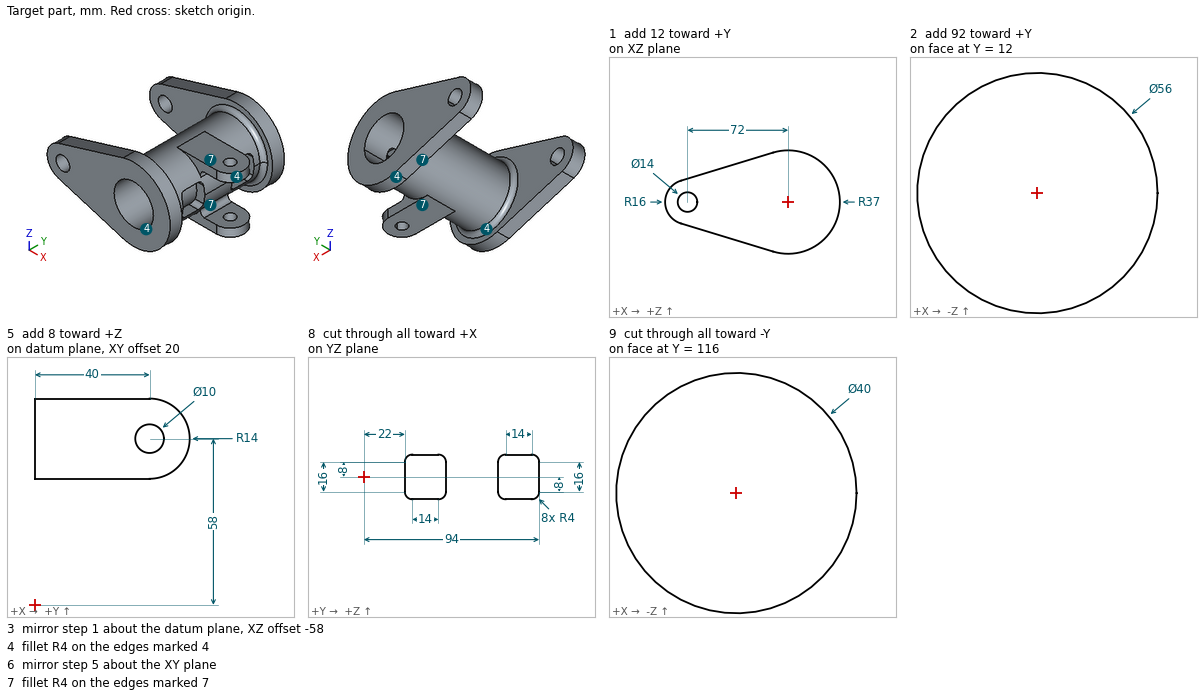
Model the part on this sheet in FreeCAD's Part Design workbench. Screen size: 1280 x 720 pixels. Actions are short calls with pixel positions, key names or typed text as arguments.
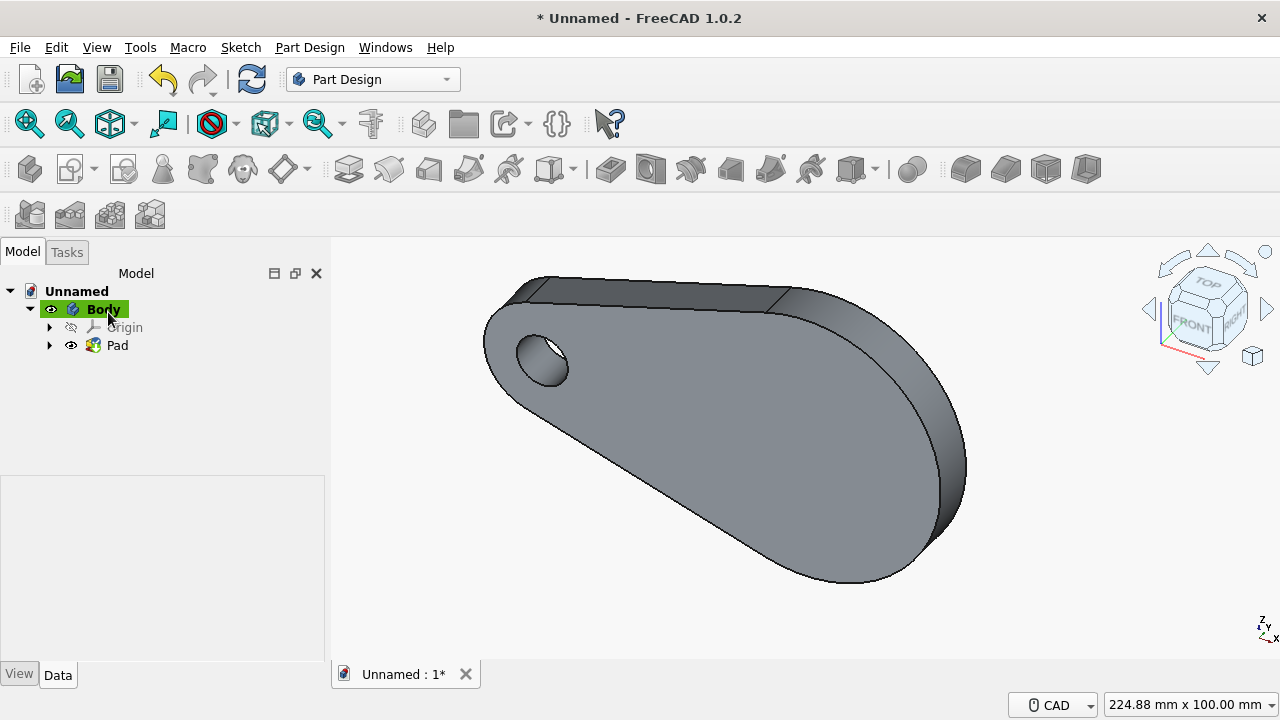
click(30, 124)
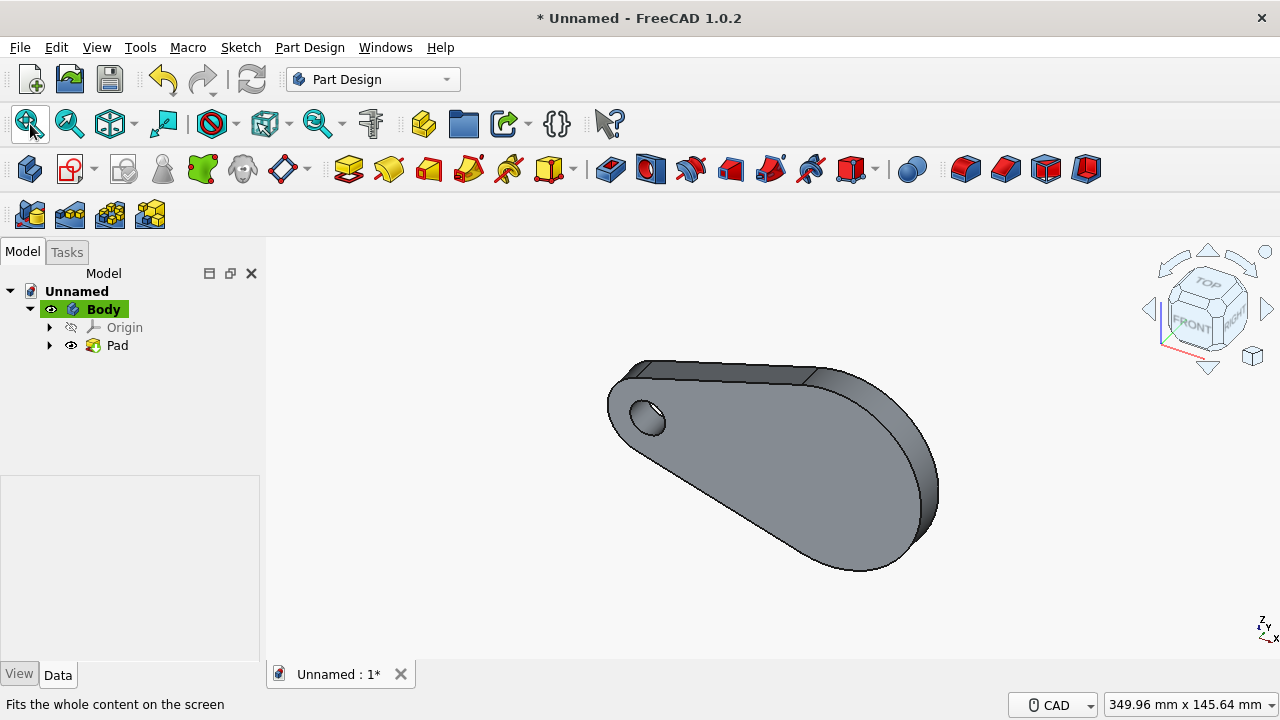
key(4)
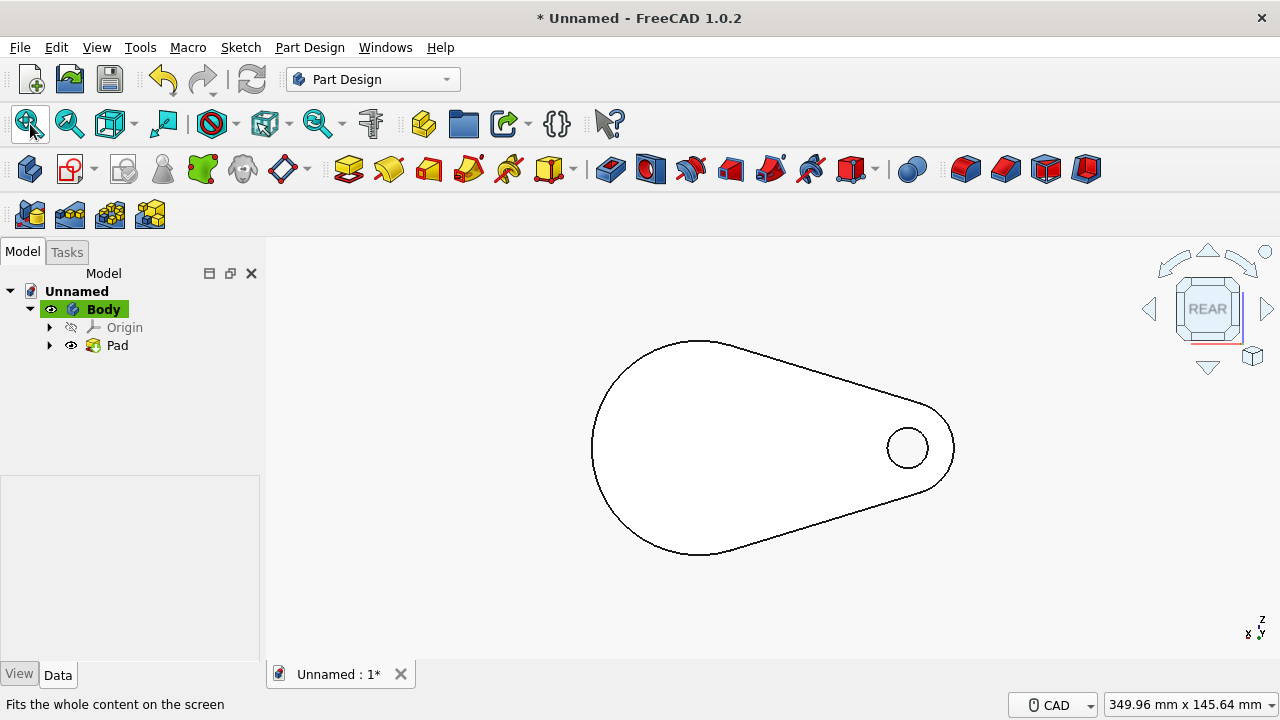
click(721, 447)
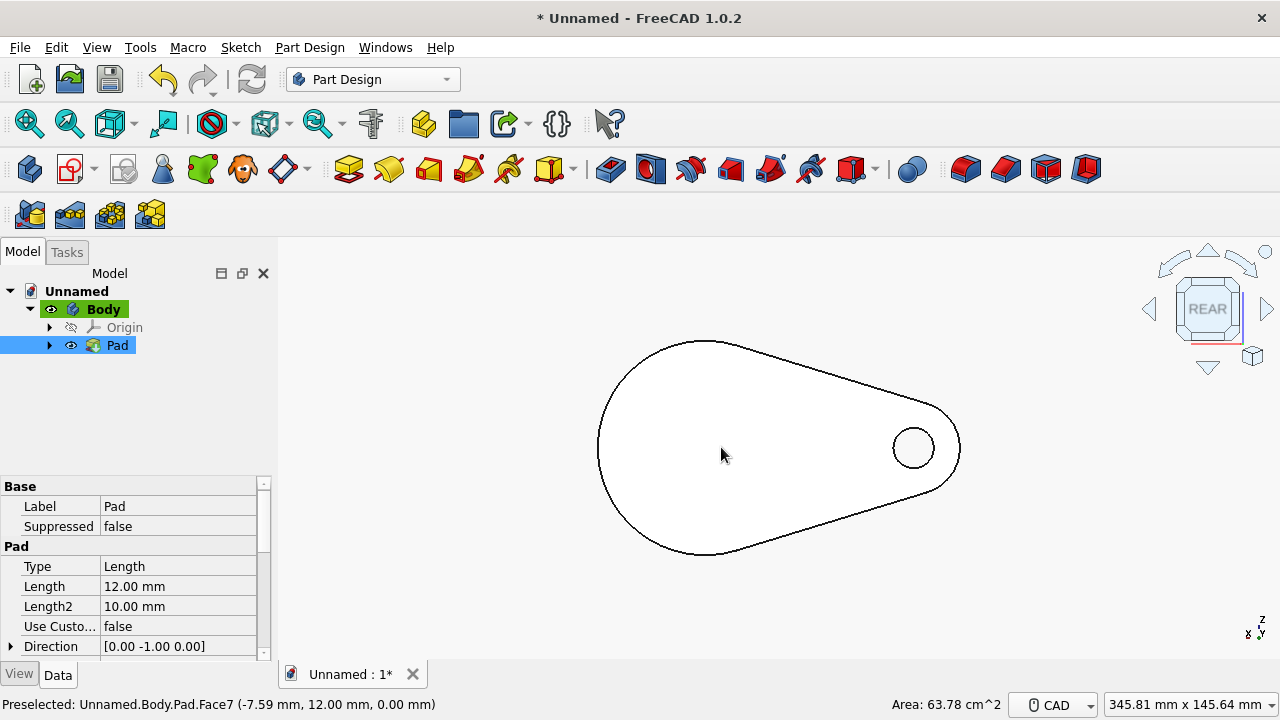
click(70, 170)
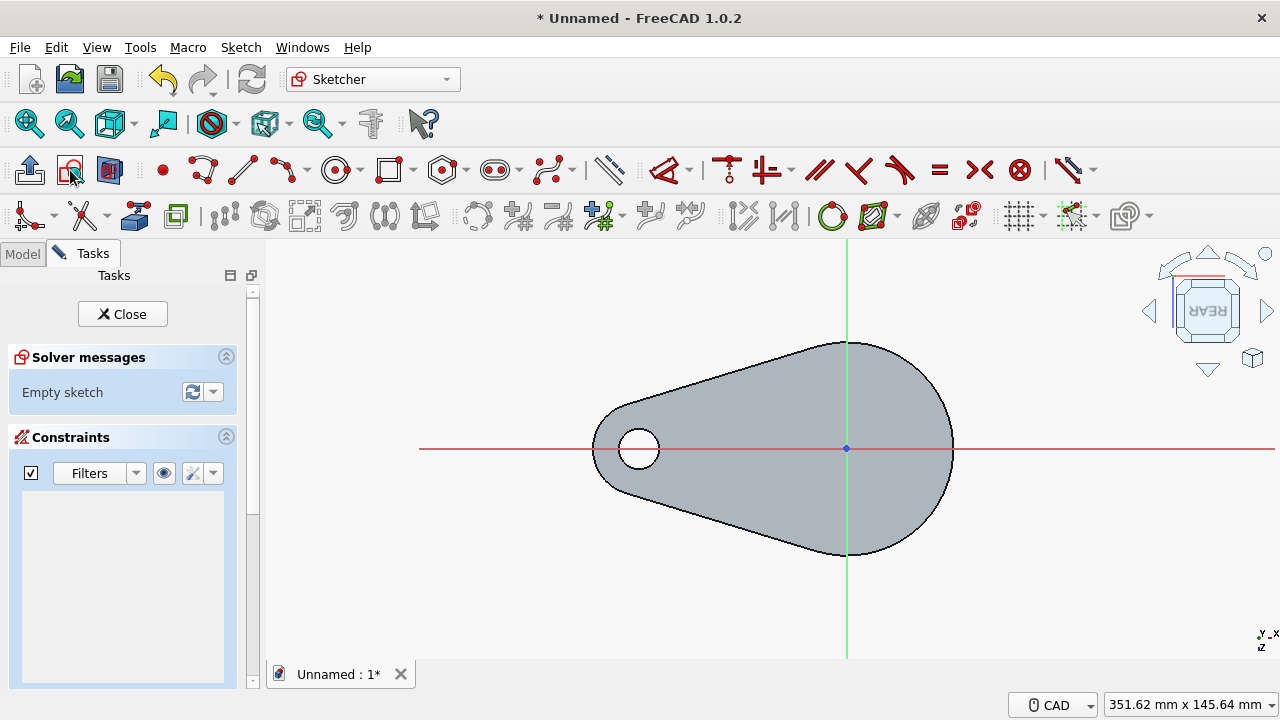
scroll(1115, 449, up, 2)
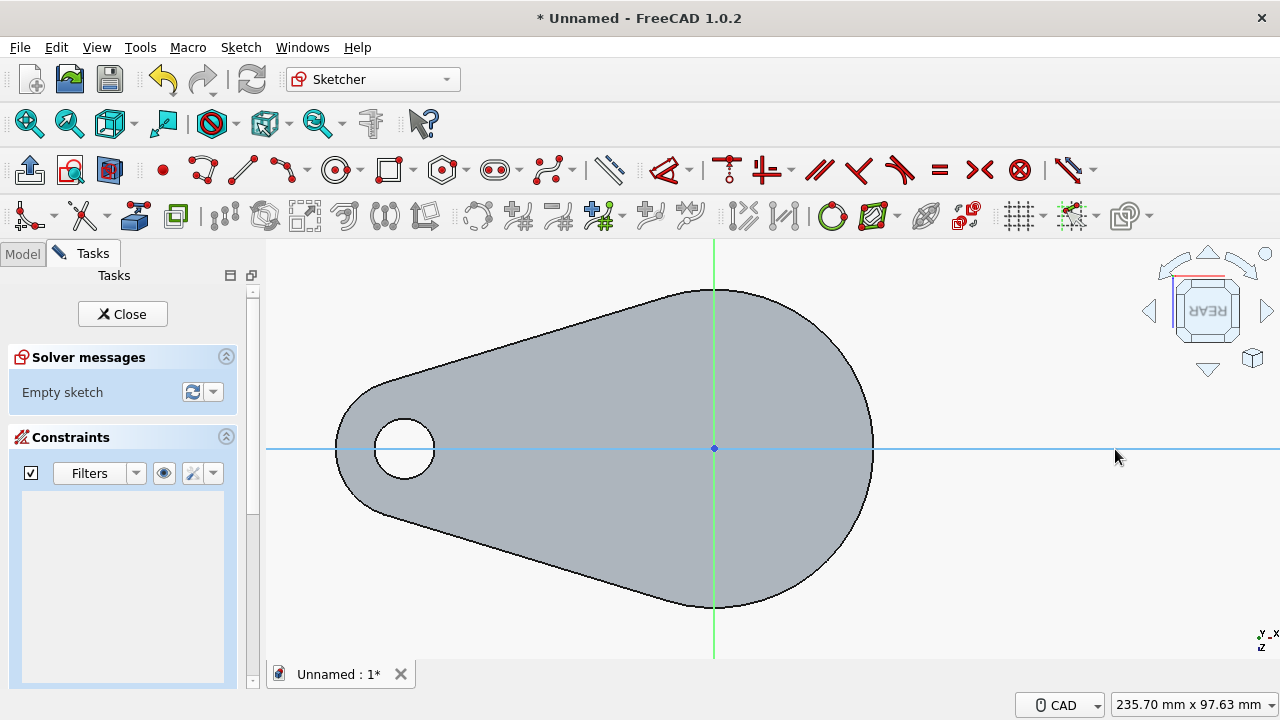
click(336, 170)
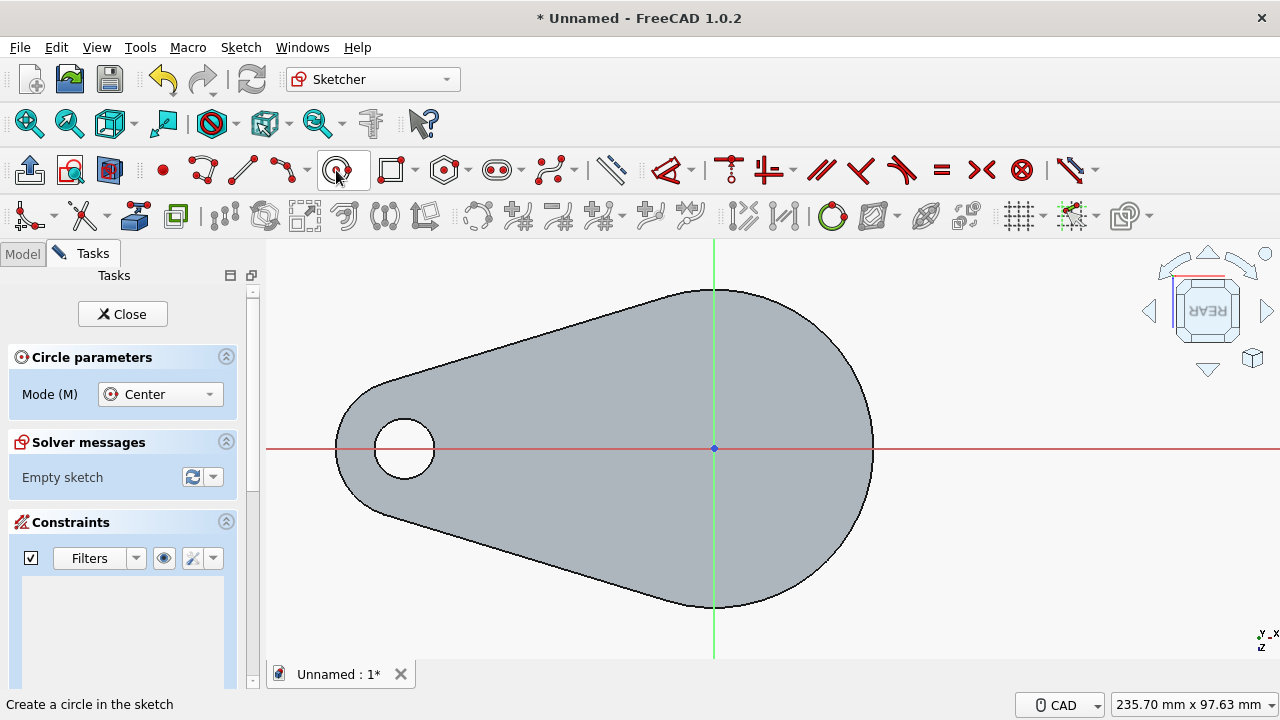
click(714, 449)
move(799, 364)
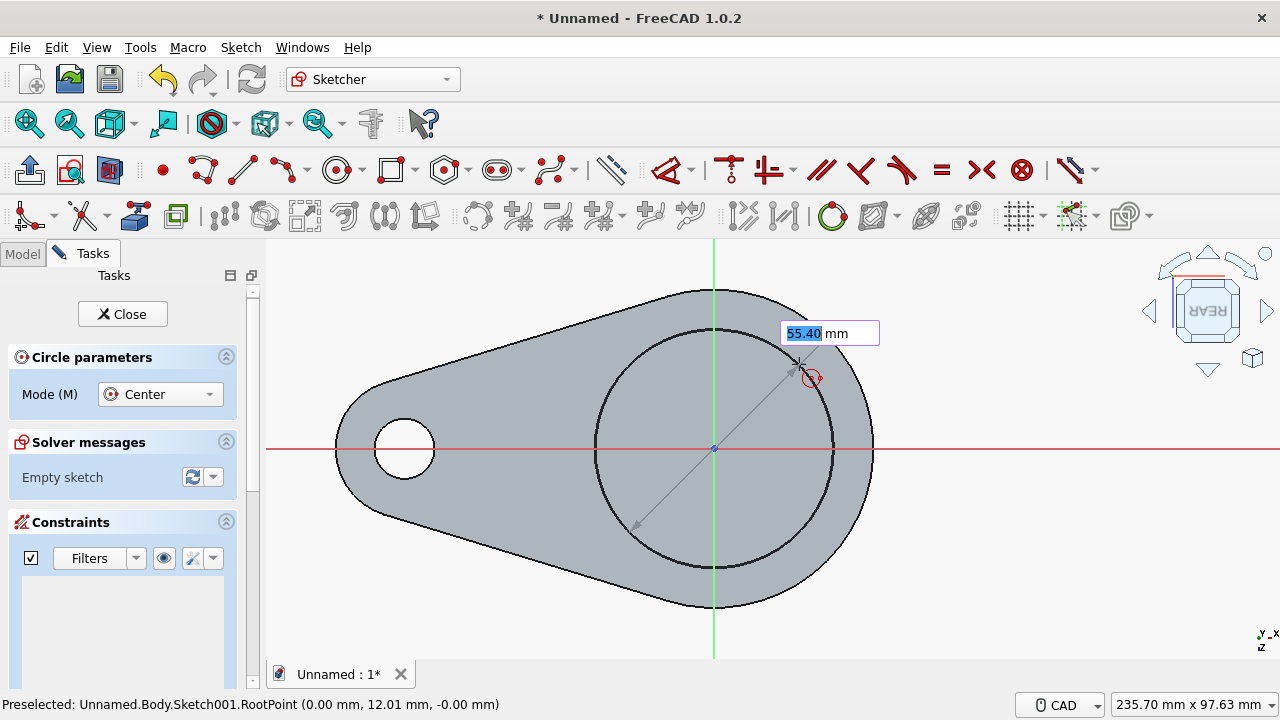
text(56)
key(Return)
key(Escape)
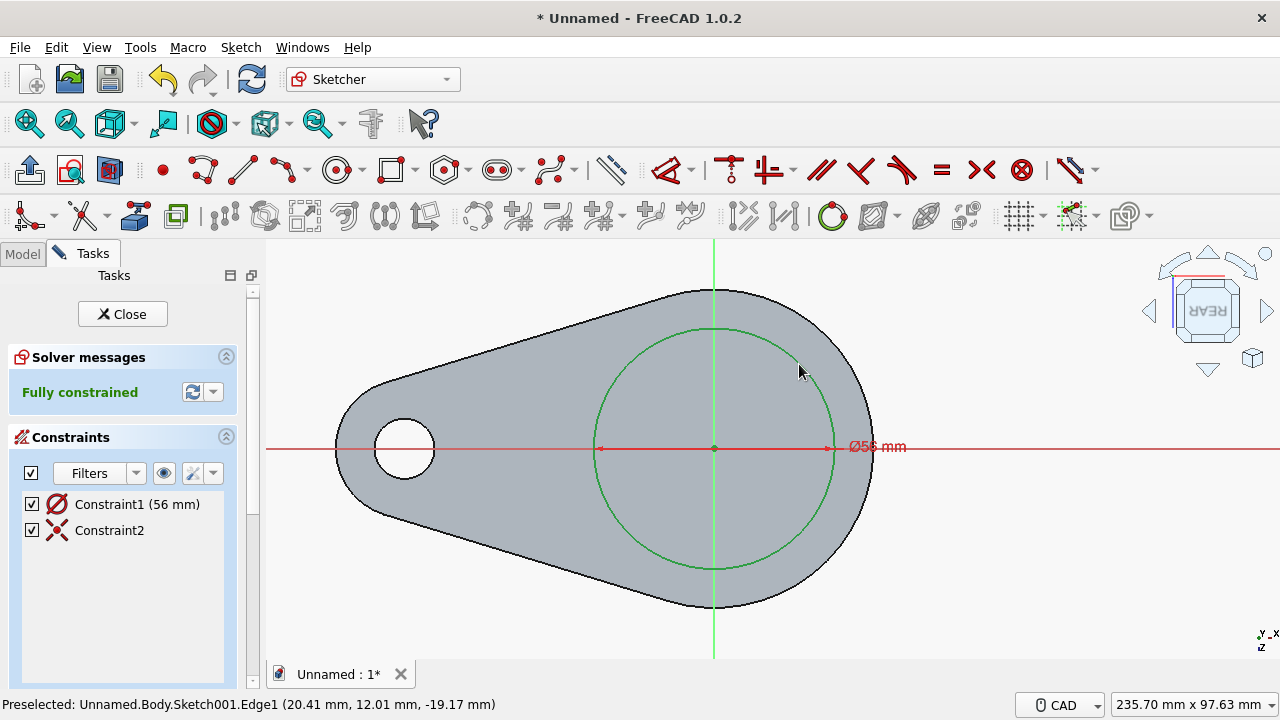
click(123, 314)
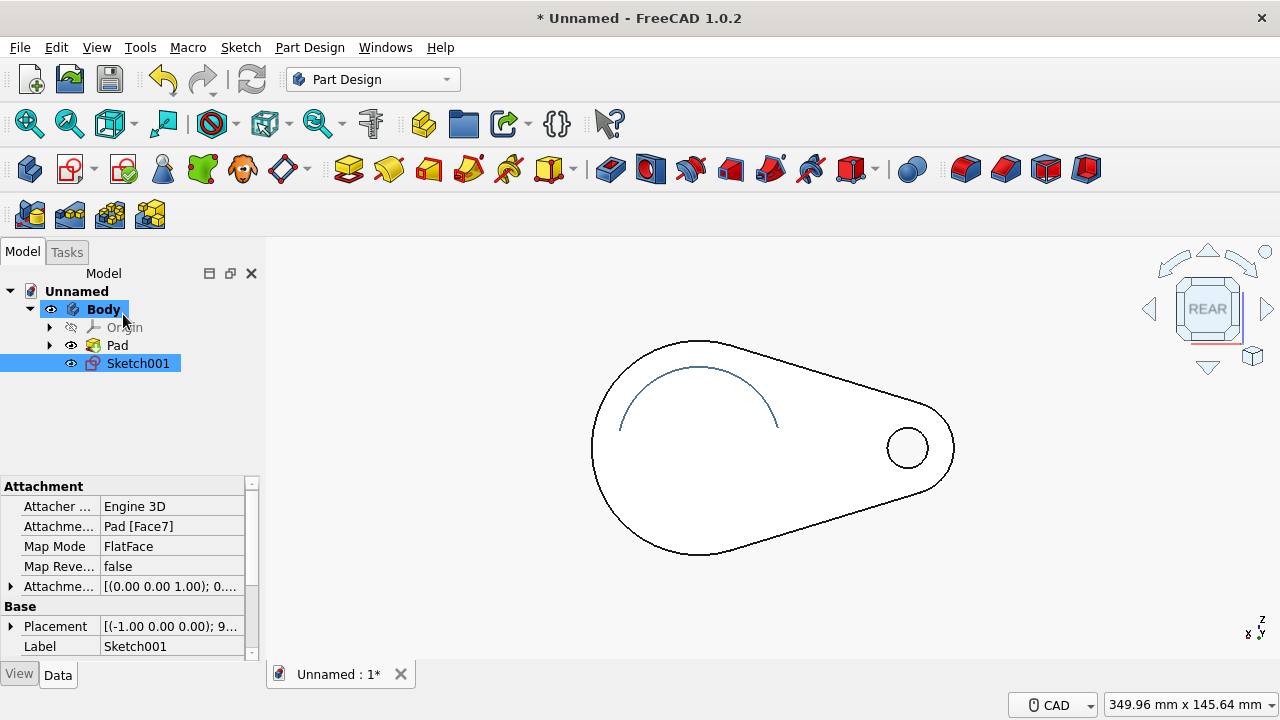
click(350, 170)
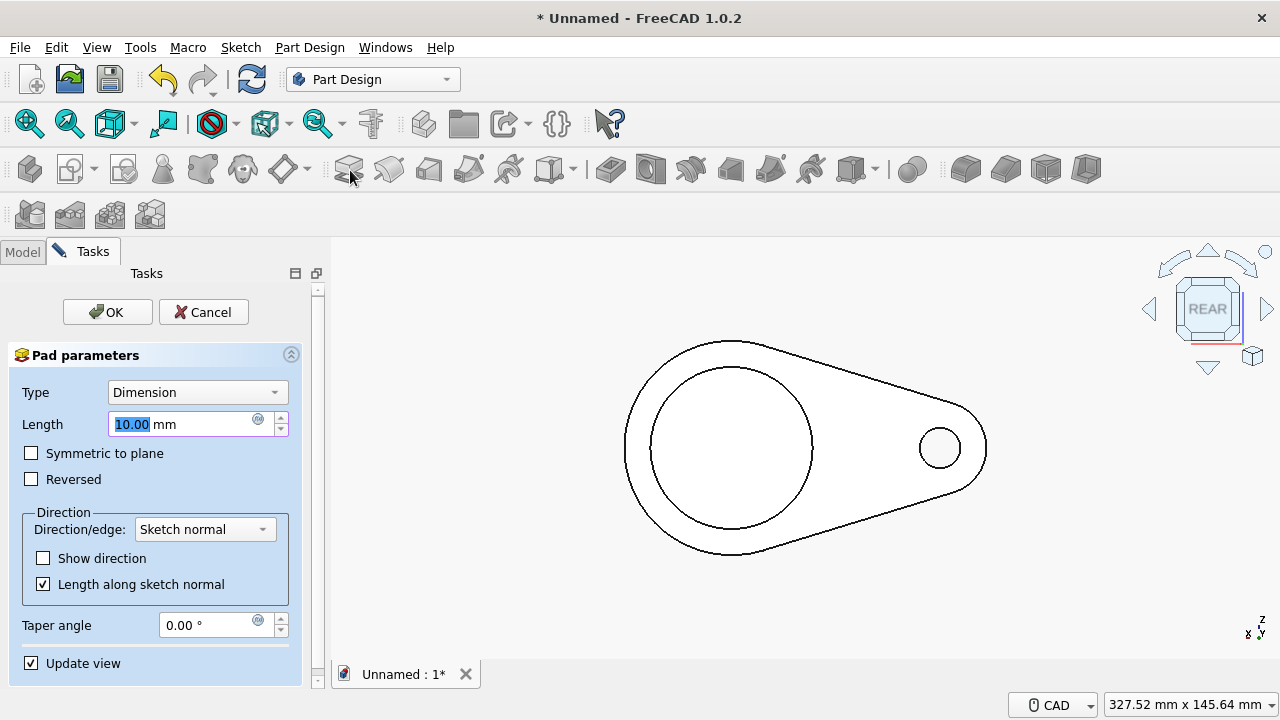
text(92)
key(Tab)